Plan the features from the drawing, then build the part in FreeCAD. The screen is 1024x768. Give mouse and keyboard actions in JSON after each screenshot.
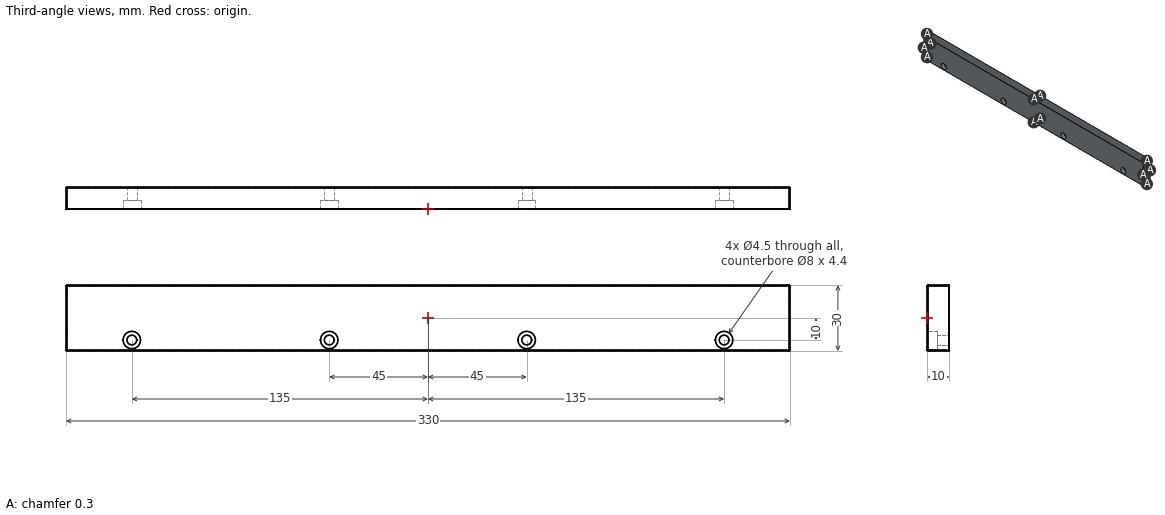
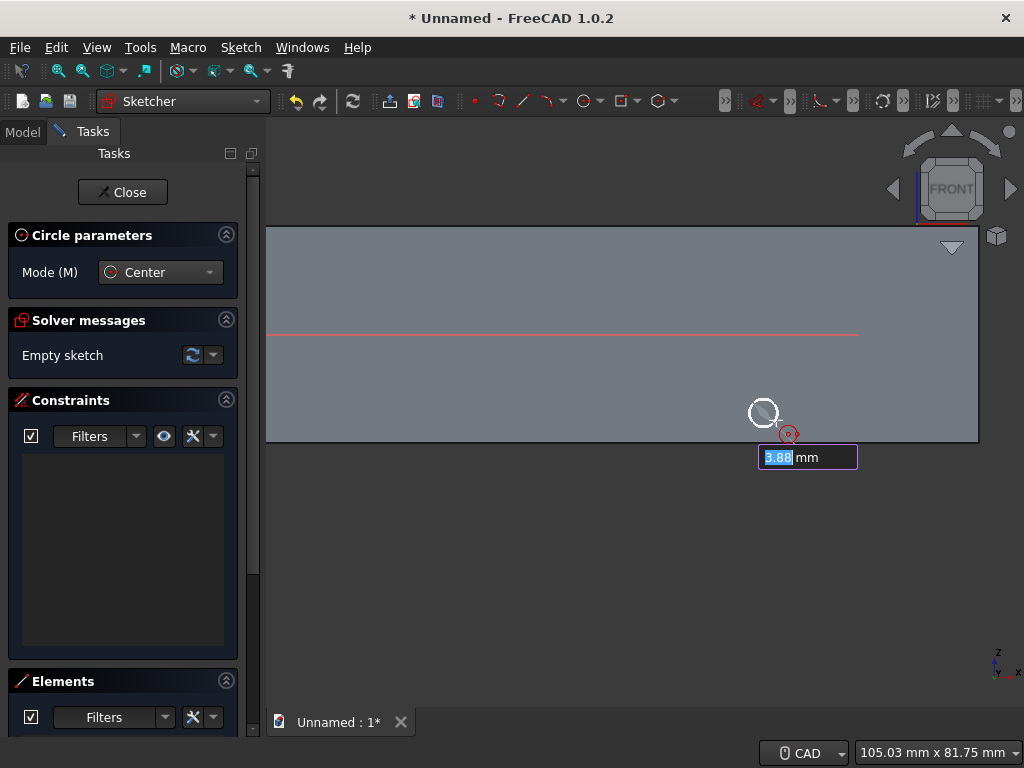
{"action": "left_click", "coordinate": [774, 418]}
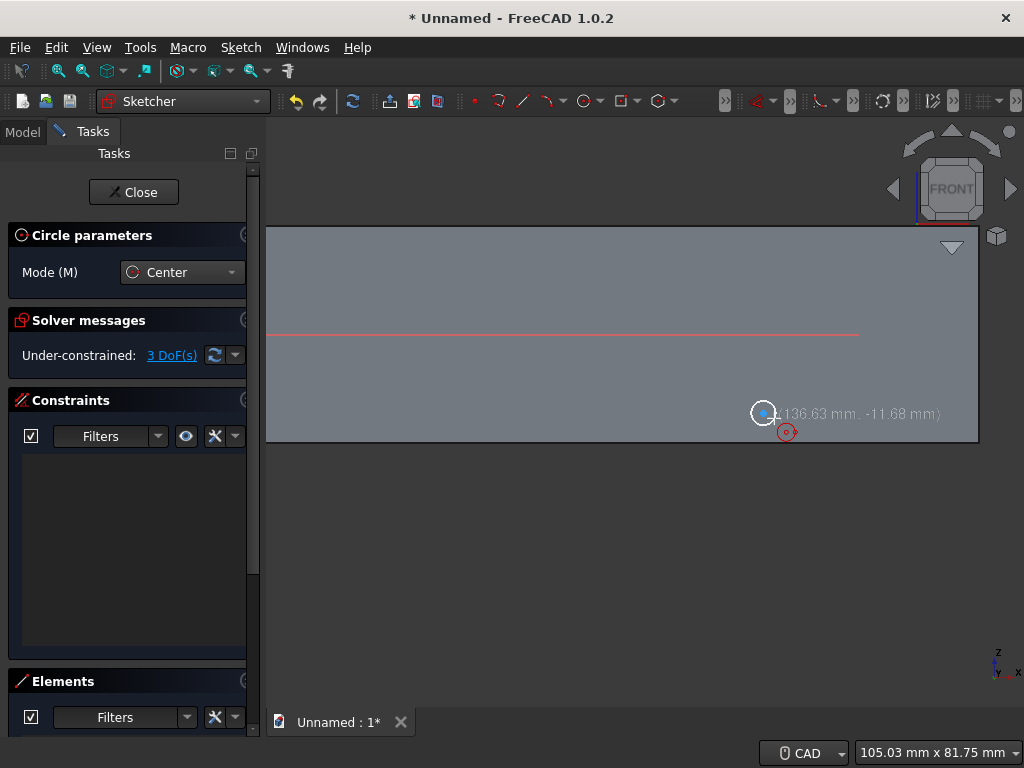
{"action": "scroll", "coordinate": [776, 420], "scroll_direction": "down", "scroll_amount": 8}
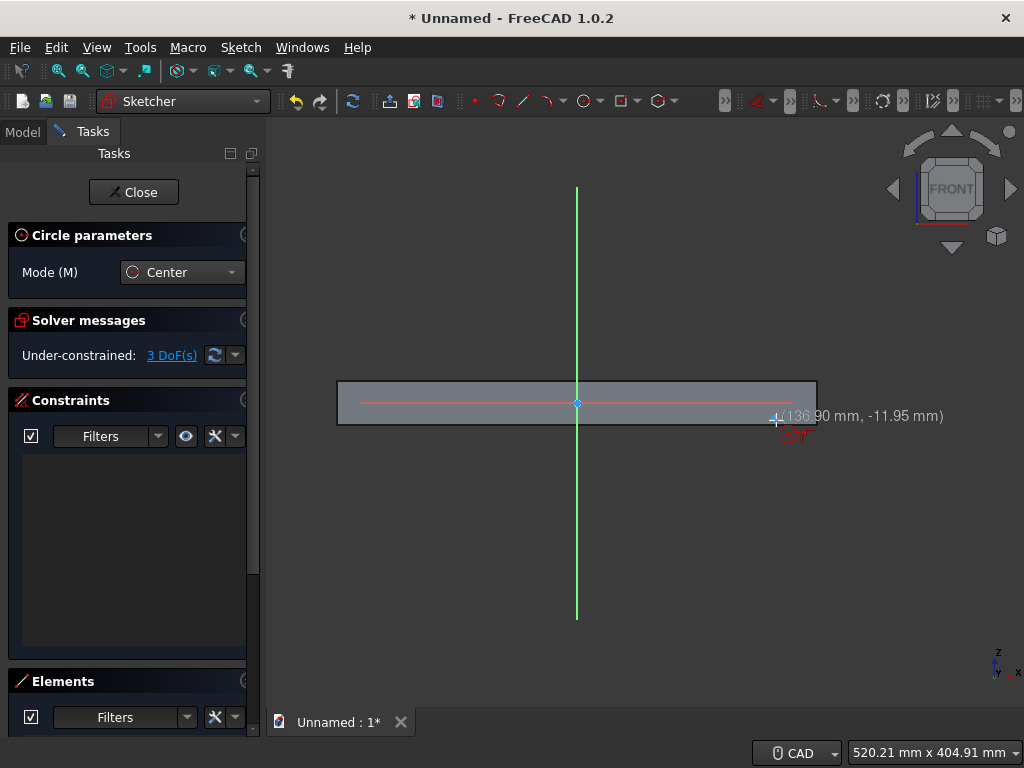
{"action": "scroll", "coordinate": [643, 418], "scroll_direction": "up", "scroll_amount": 10}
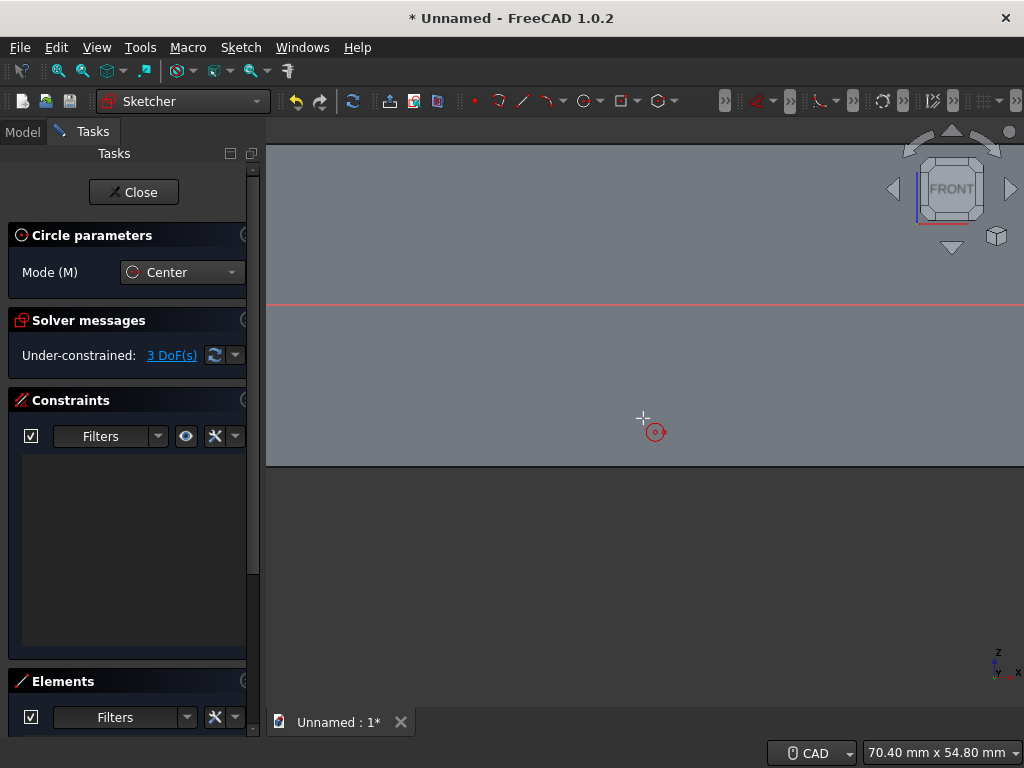
{"action": "scroll", "coordinate": [643, 418], "scroll_direction": "down", "scroll_amount": 10}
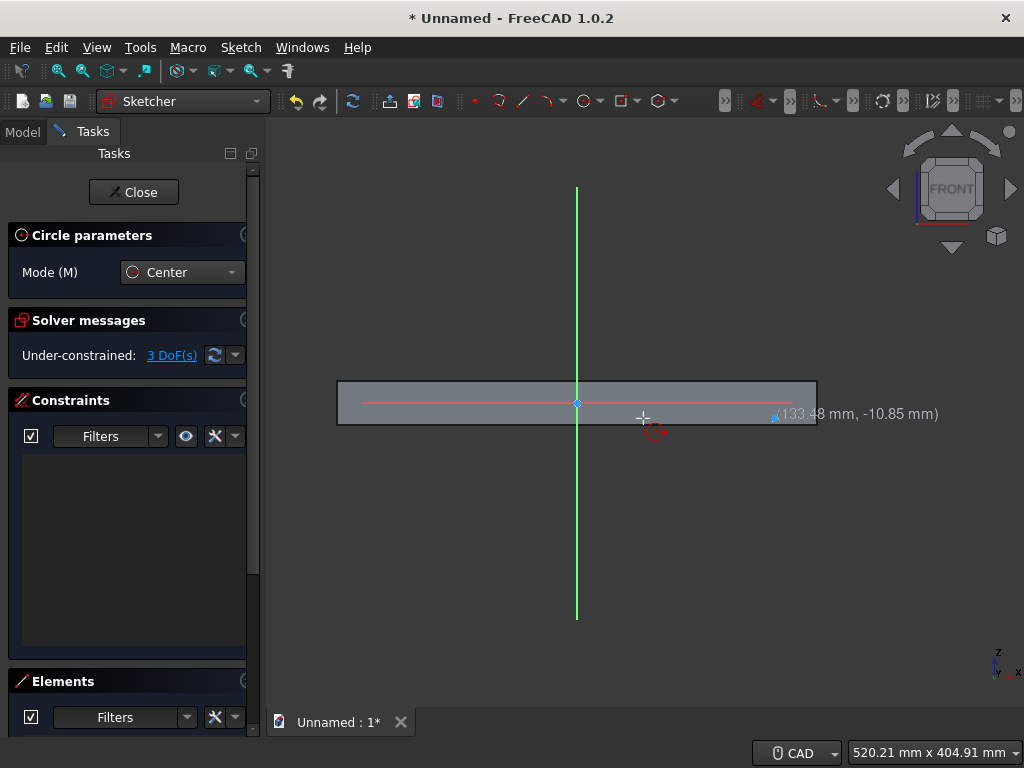
{"action": "left_click", "coordinate": [643, 418]}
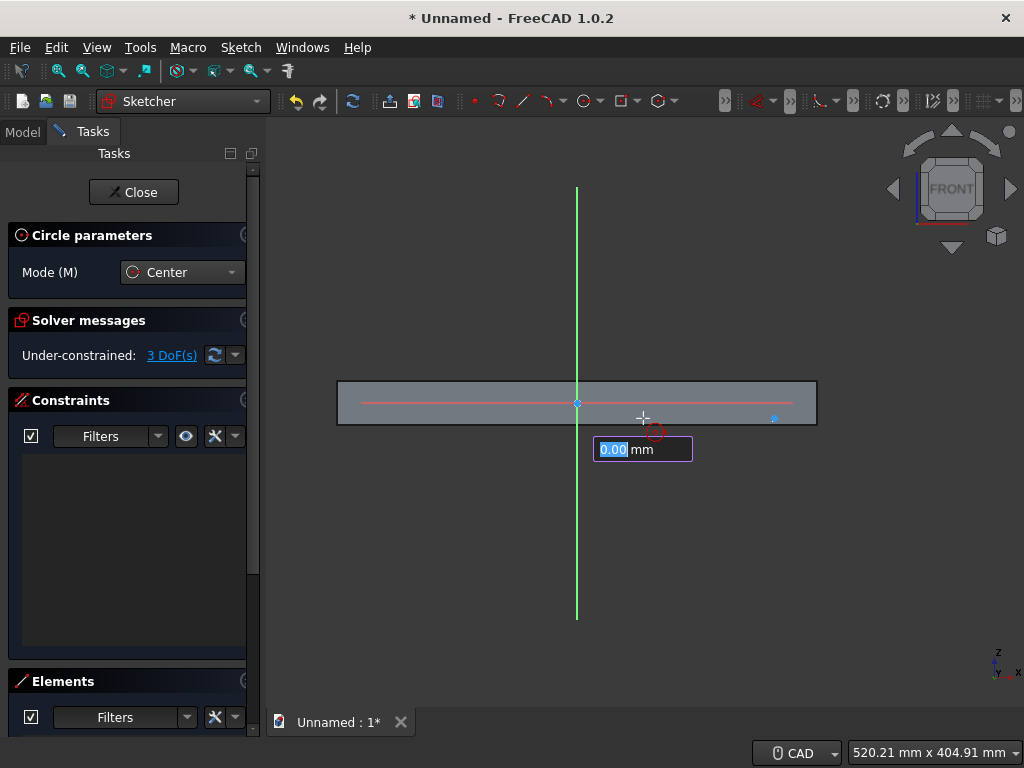
{"action": "scroll", "coordinate": [645, 420], "scroll_direction": "up", "scroll_amount": 8}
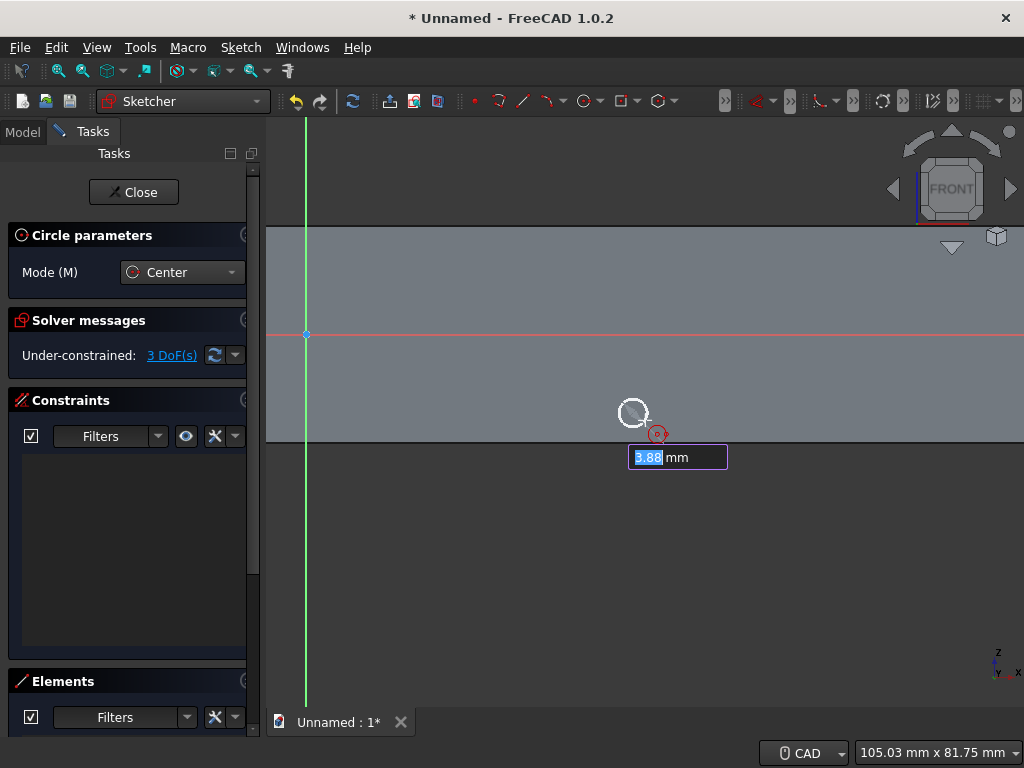
{"action": "left_click", "coordinate": [643, 418]}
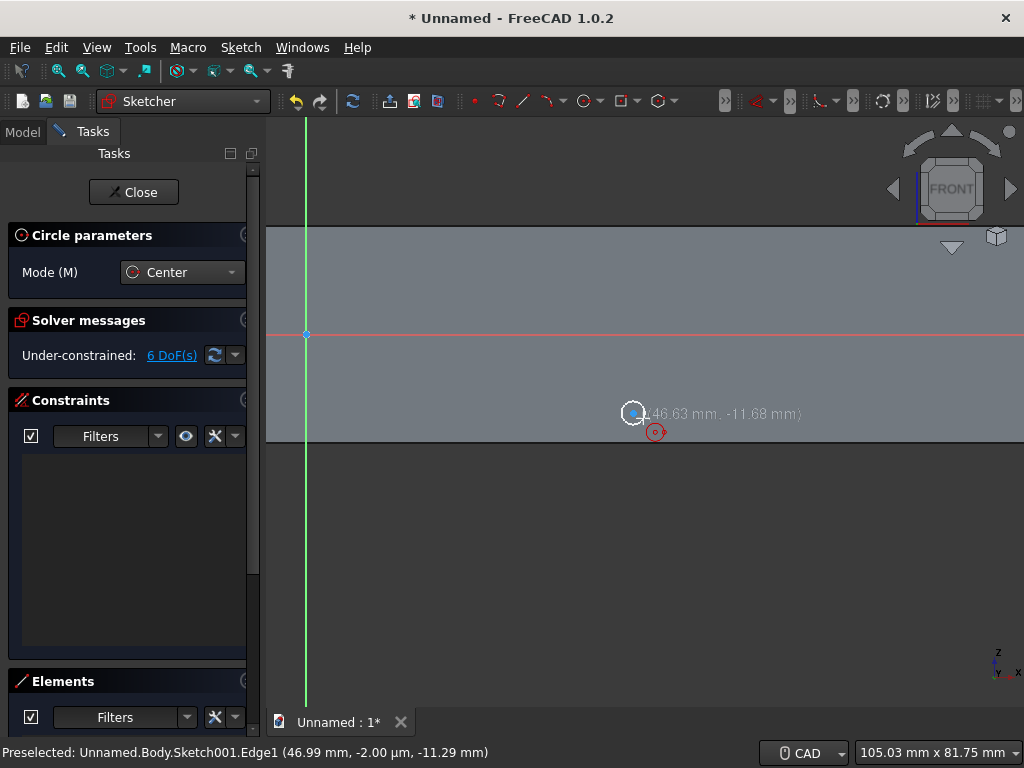
{"action": "scroll", "coordinate": [645, 420], "scroll_direction": "down", "scroll_amount": 8}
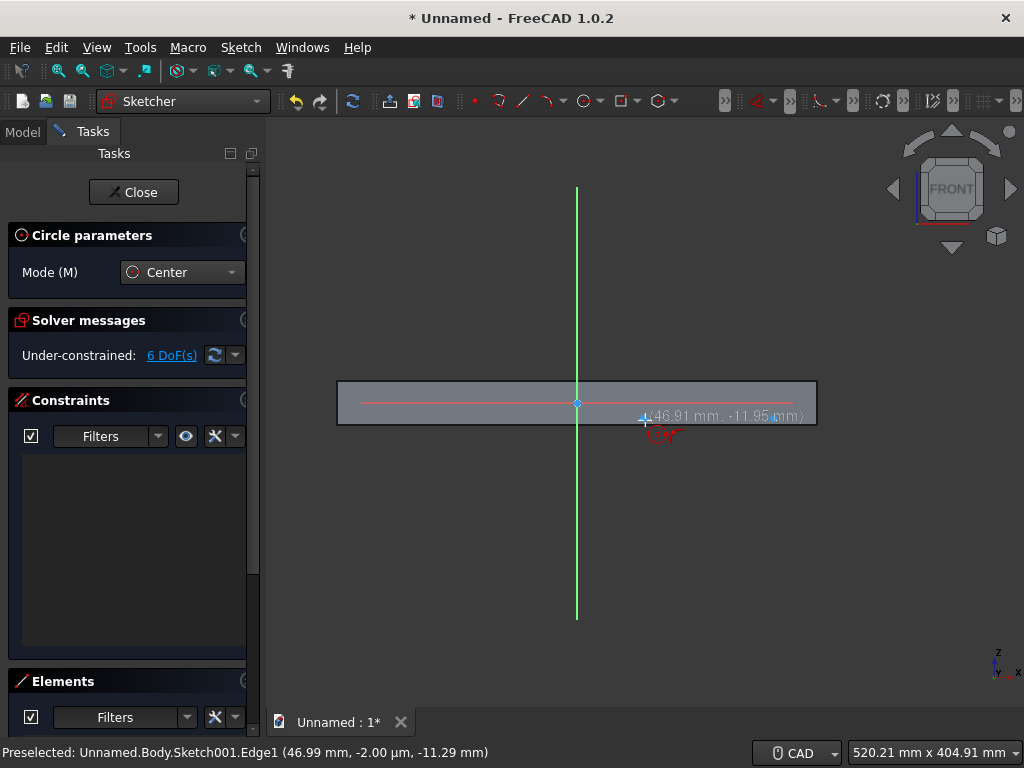
{"action": "scroll", "coordinate": [511, 418], "scroll_direction": "up", "scroll_amount": 10}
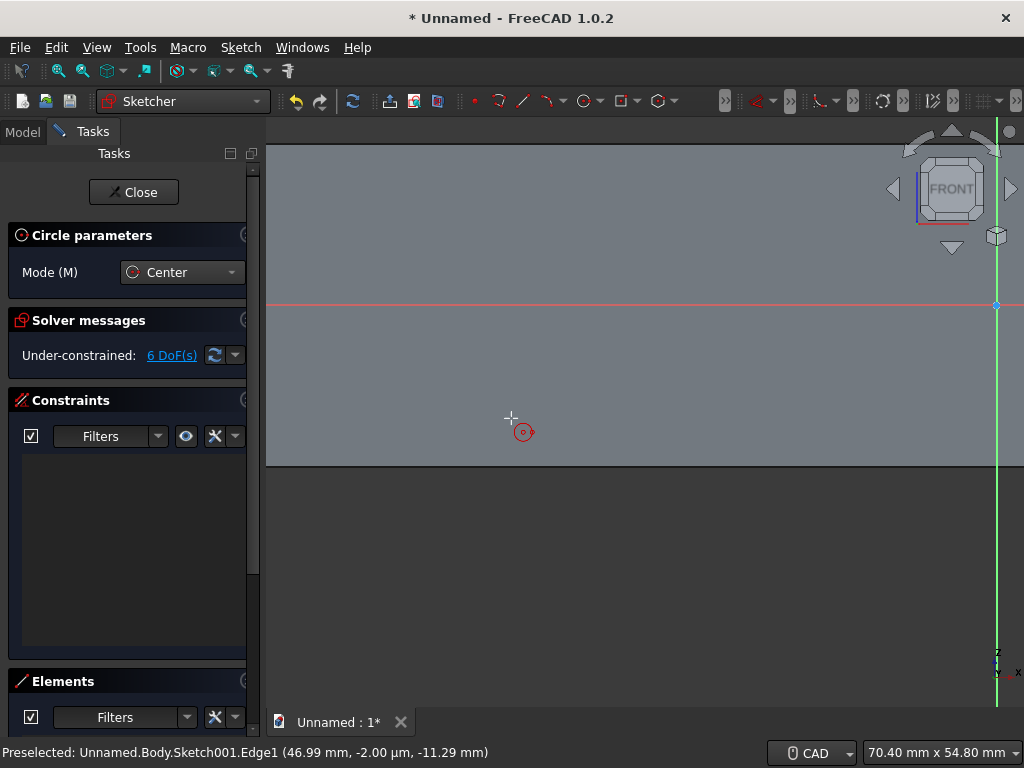
{"action": "scroll", "coordinate": [511, 418], "scroll_direction": "down", "scroll_amount": 10}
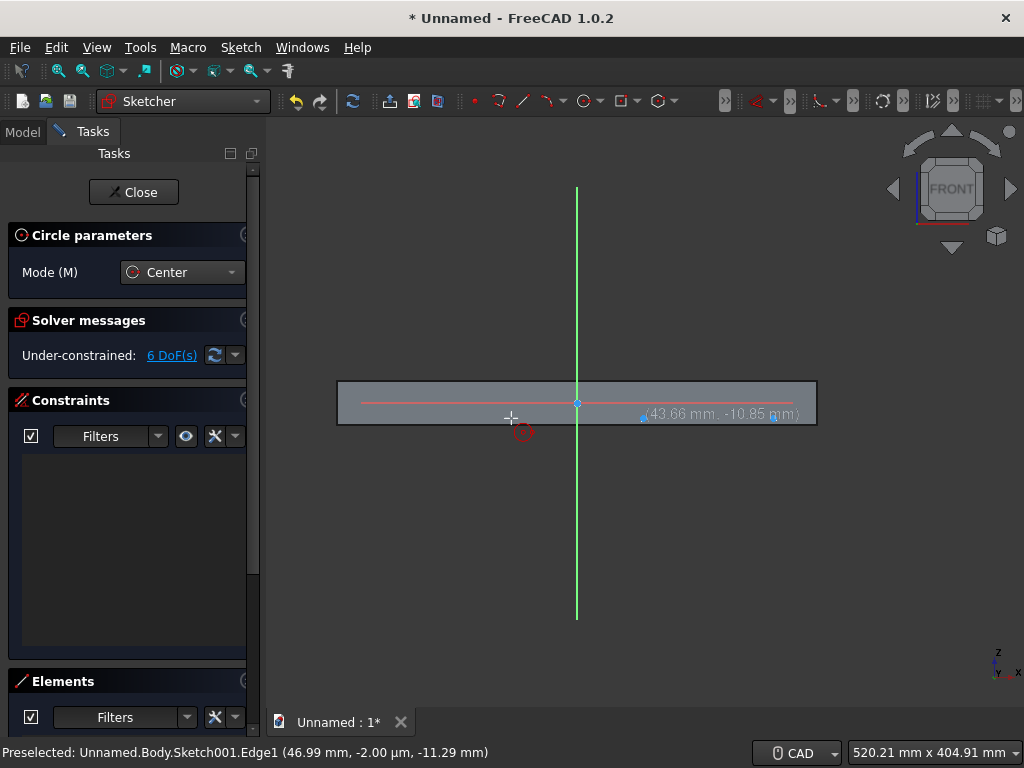
{"action": "left_click", "coordinate": [511, 418]}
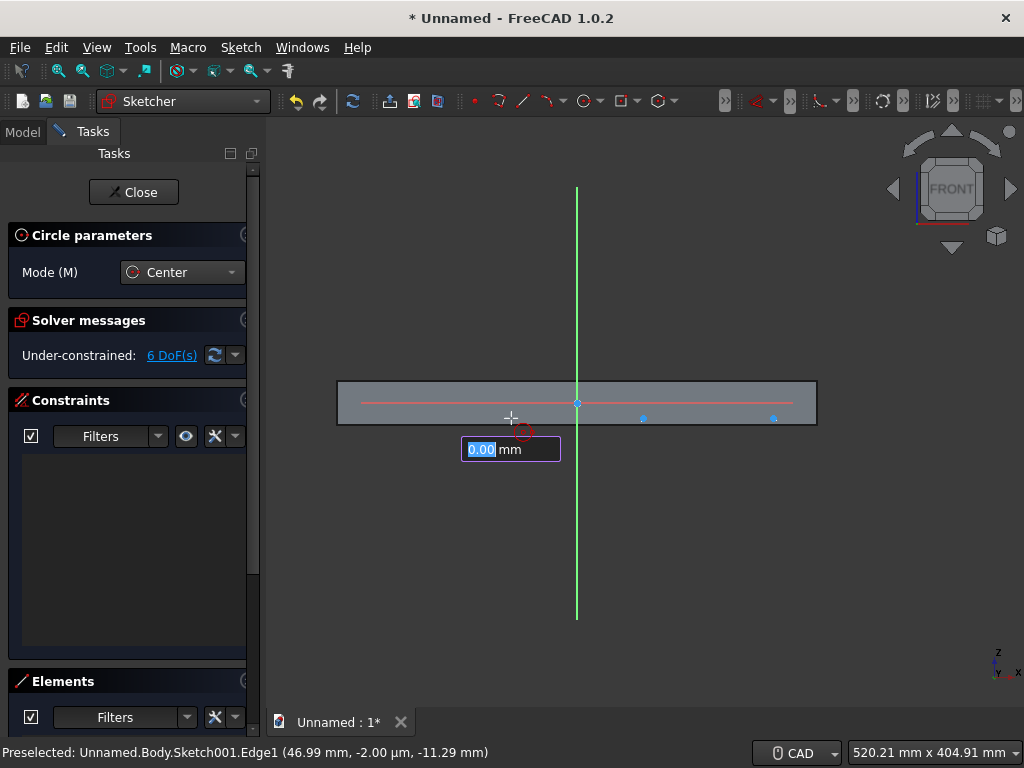
{"action": "scroll", "coordinate": [514, 420], "scroll_direction": "up", "scroll_amount": 8}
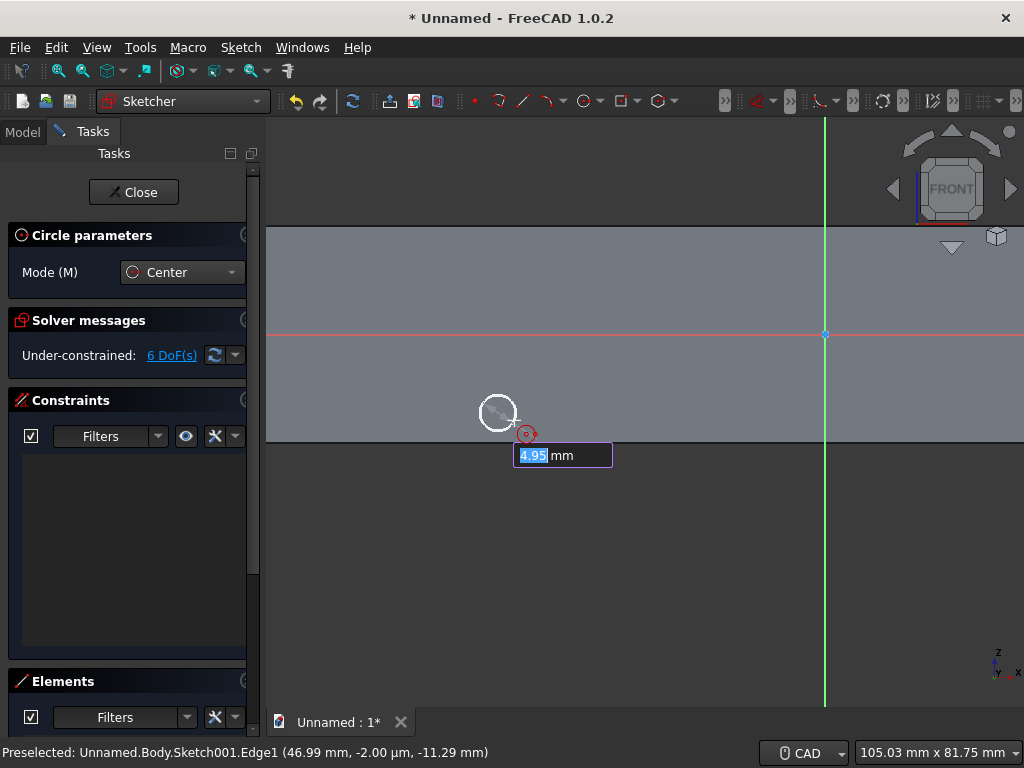
{"action": "left_click", "coordinate": [512, 418]}